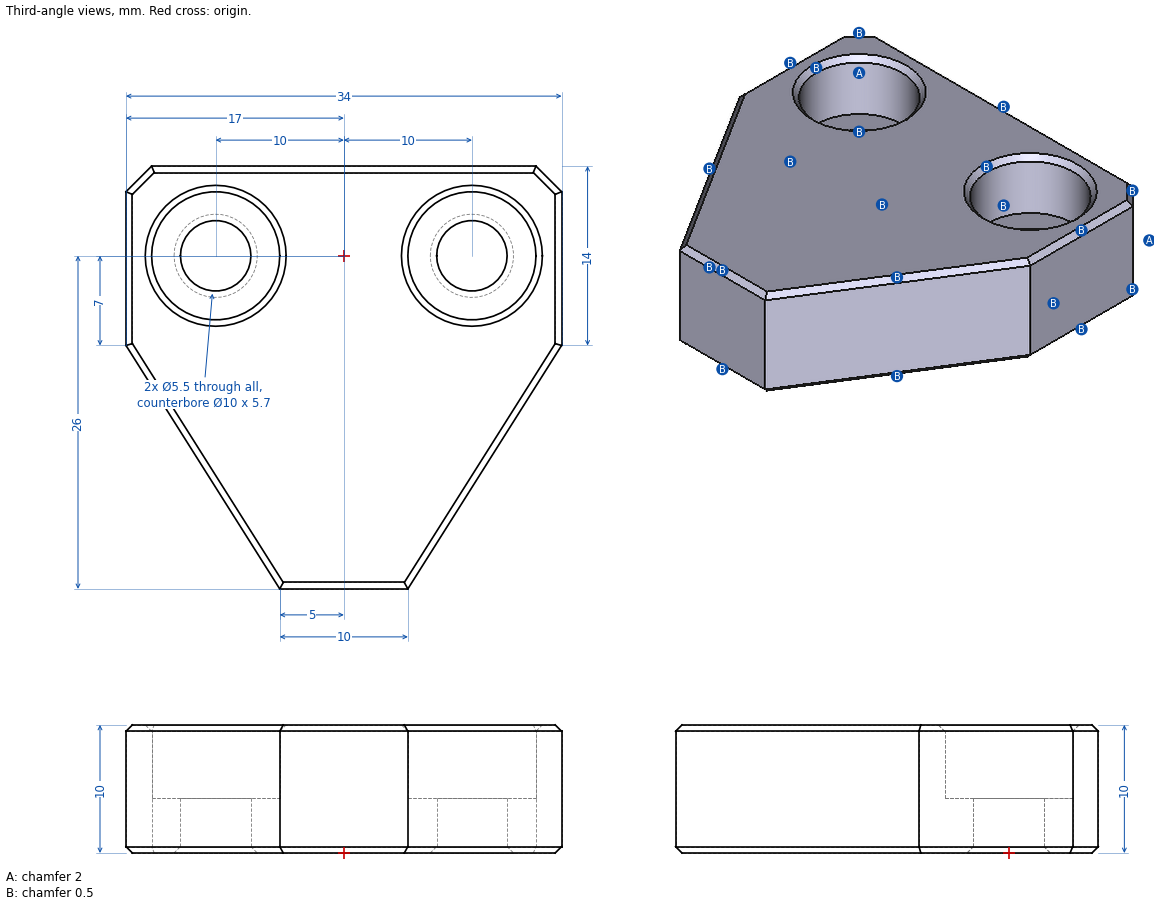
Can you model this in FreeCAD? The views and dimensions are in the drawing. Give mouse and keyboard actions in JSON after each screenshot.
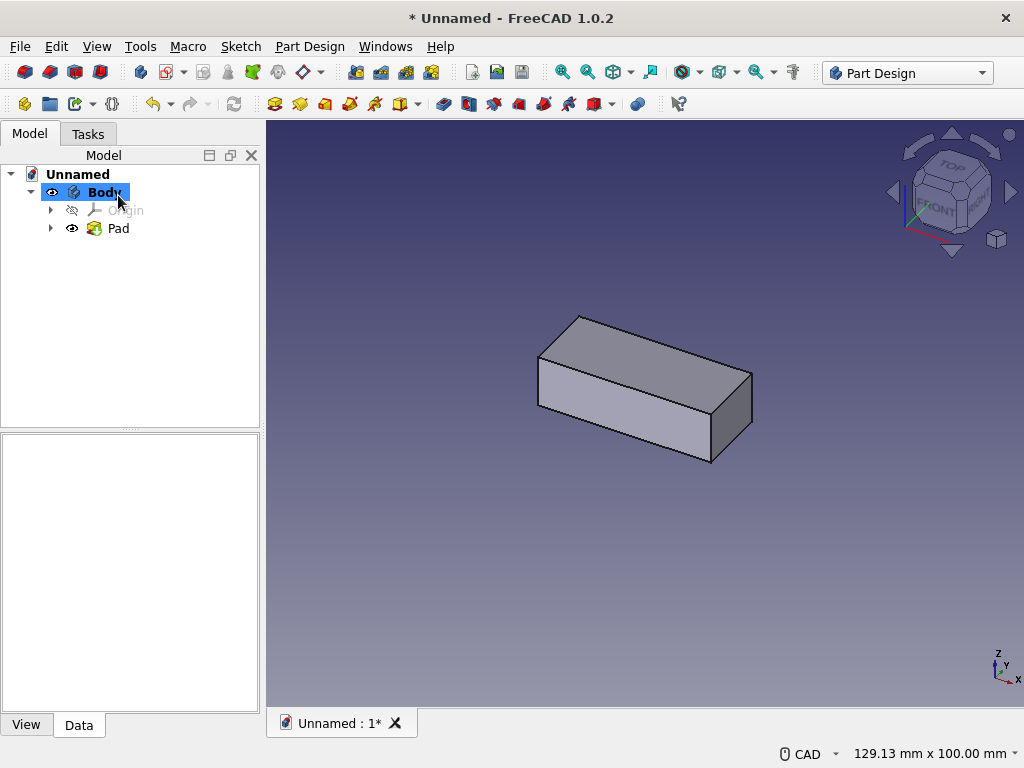
{"action": "left_click", "coordinate": [563, 72]}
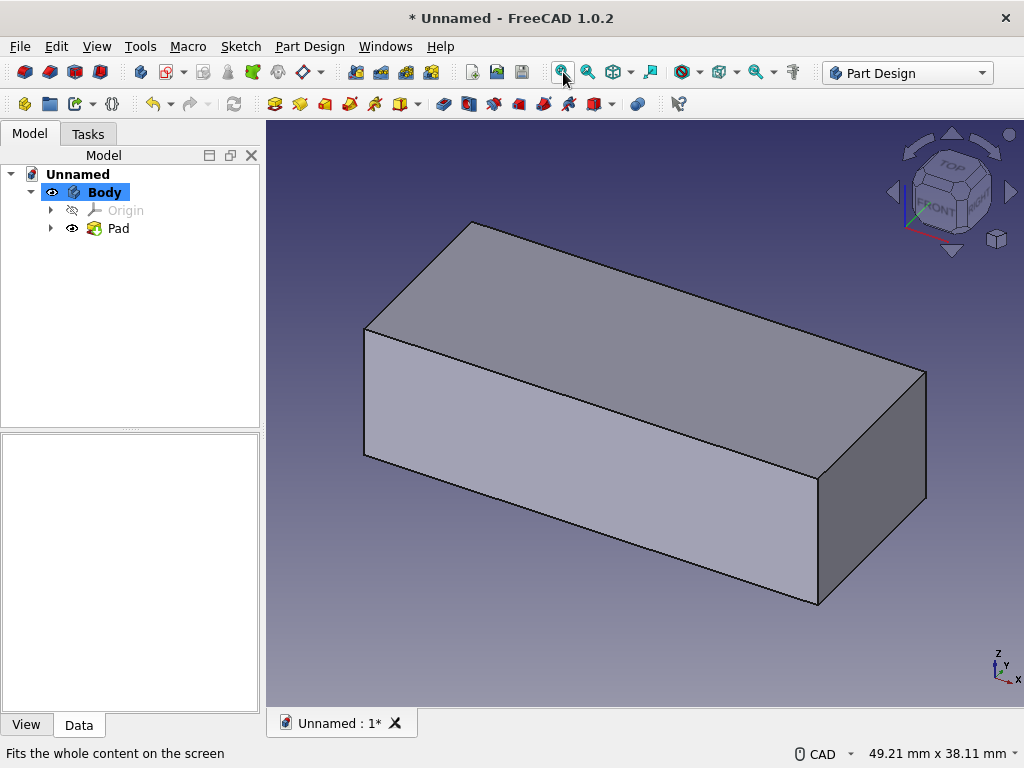
{"action": "left_click", "coordinate": [775, 392]}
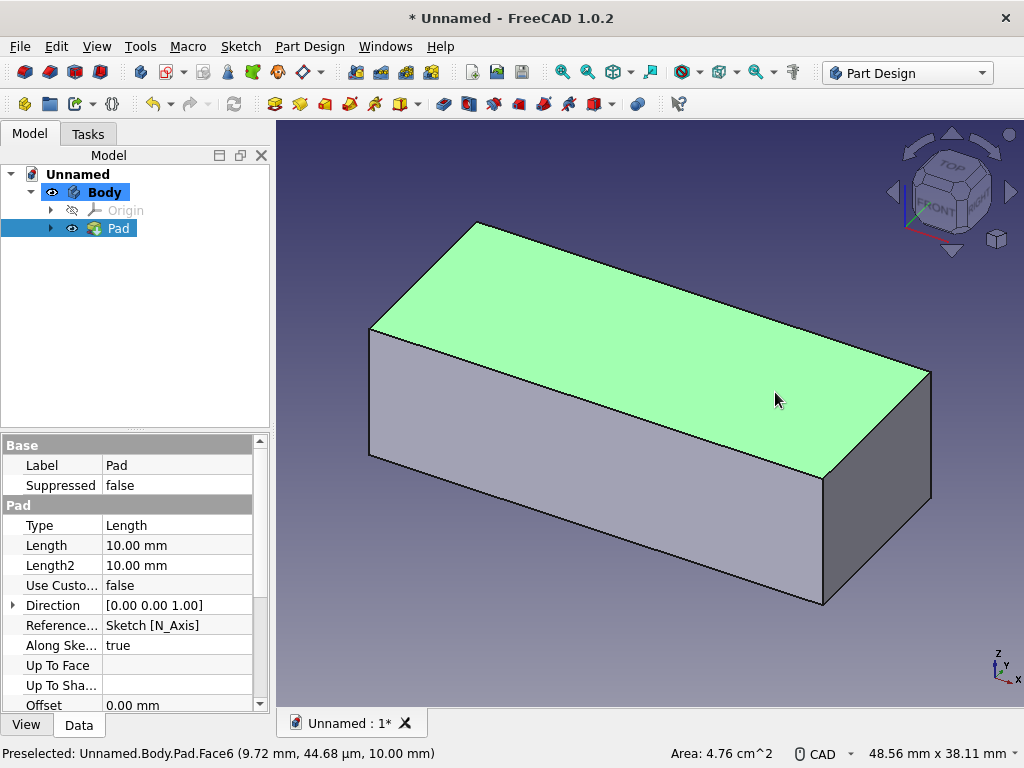
{"action": "left_click", "coordinate": [166, 72]}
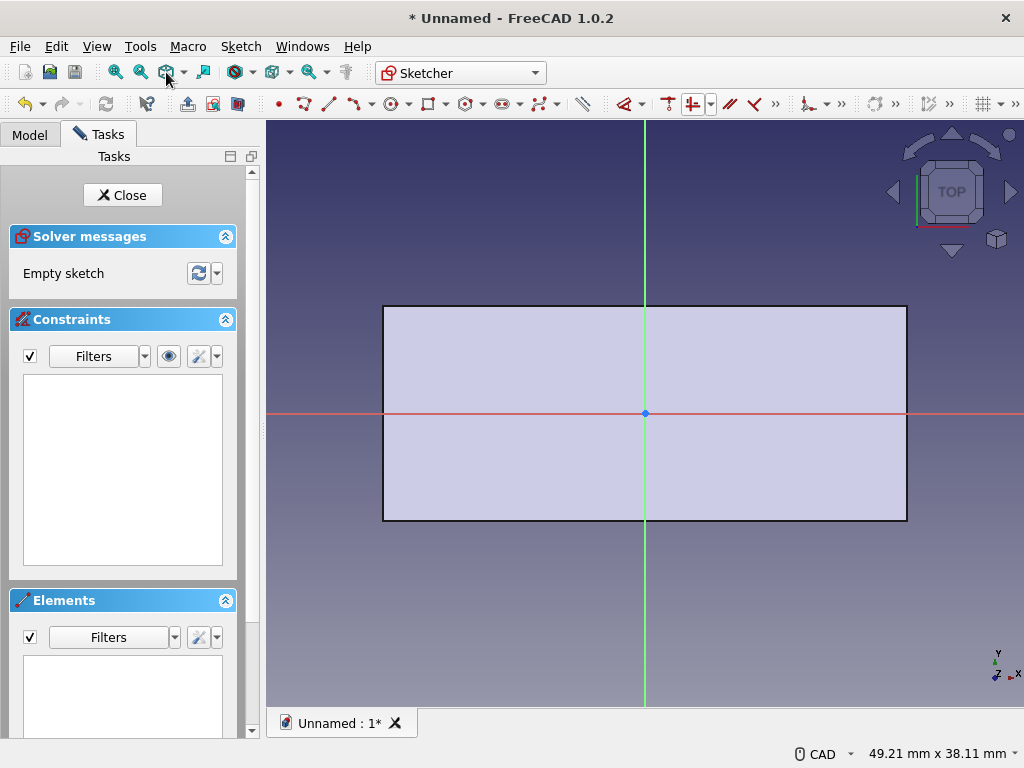
{"action": "scroll", "coordinate": [294, 413], "scroll_direction": "down", "scroll_amount": 1}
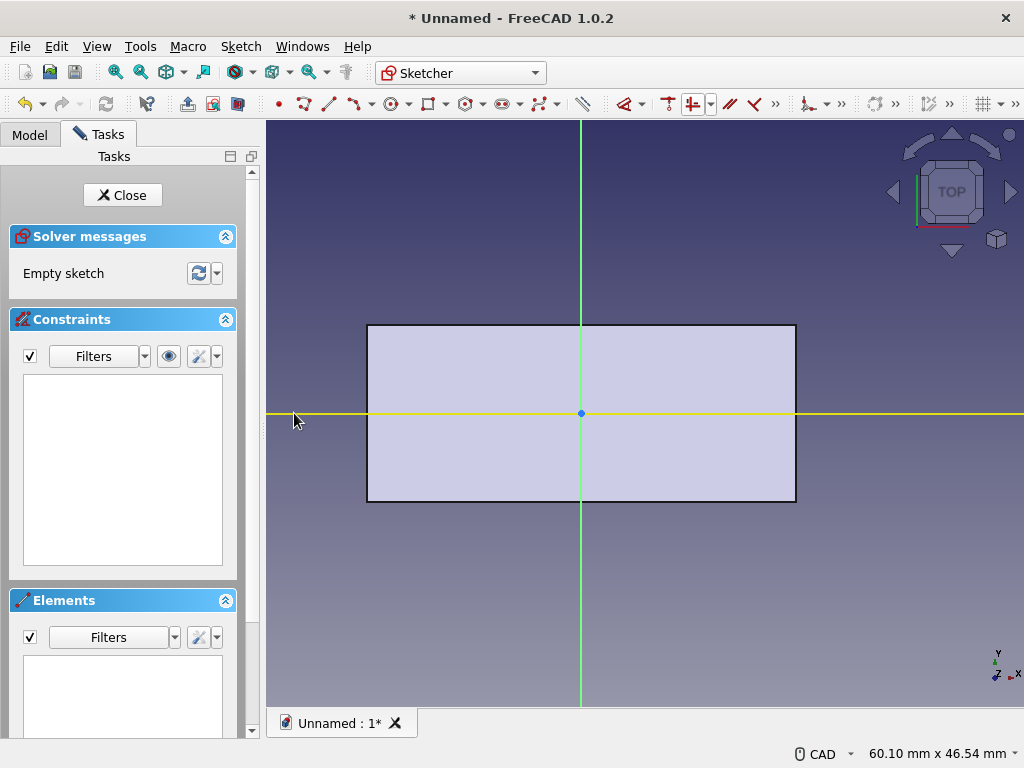
{"action": "left_click", "coordinate": [390, 104]}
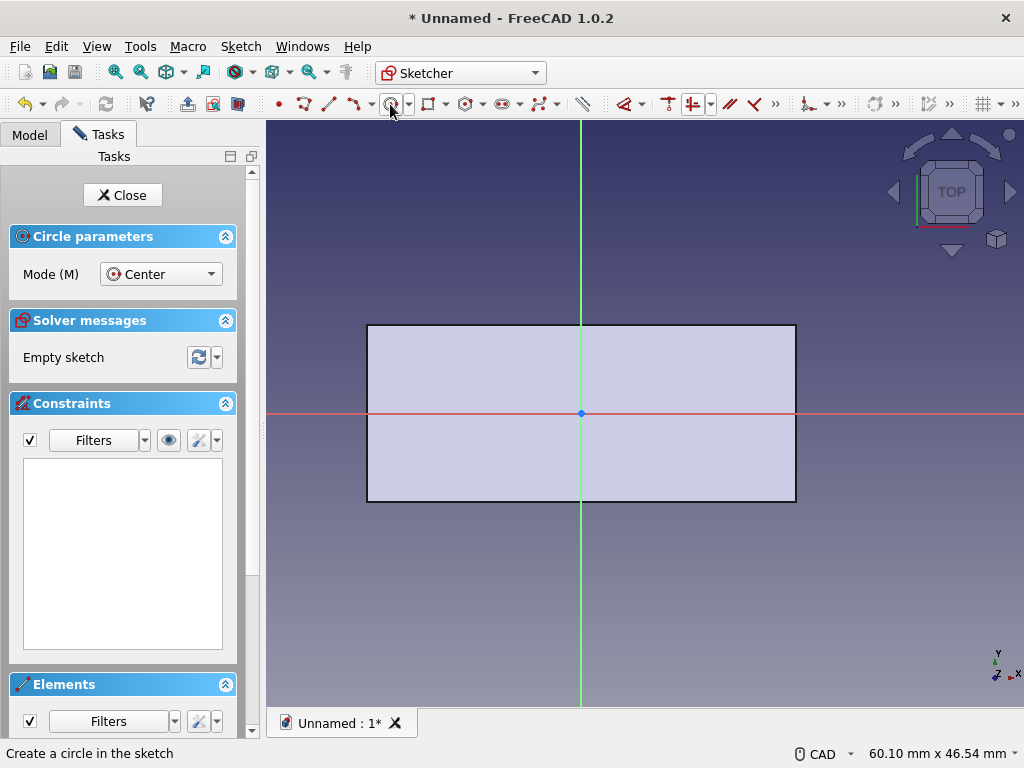
{"action": "left_click", "coordinate": [455, 414]}
{"action": "mouse_move", "coordinate": [480, 389]}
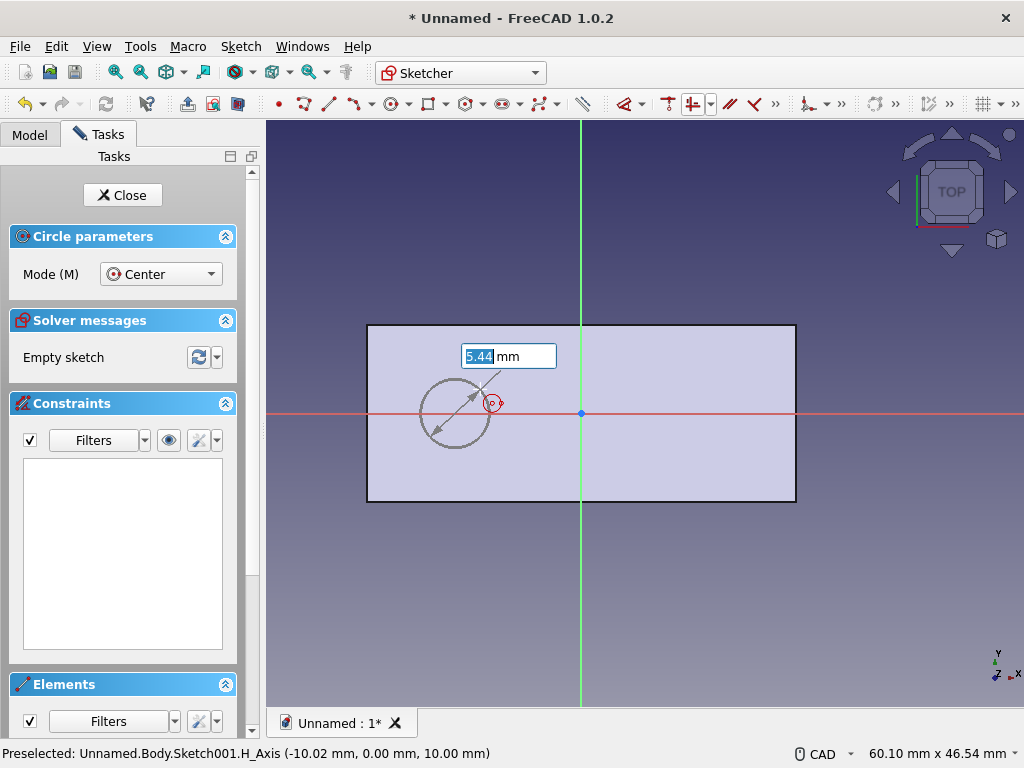
{"action": "type", "text": "5.5"}
{"action": "key", "text": "Return"}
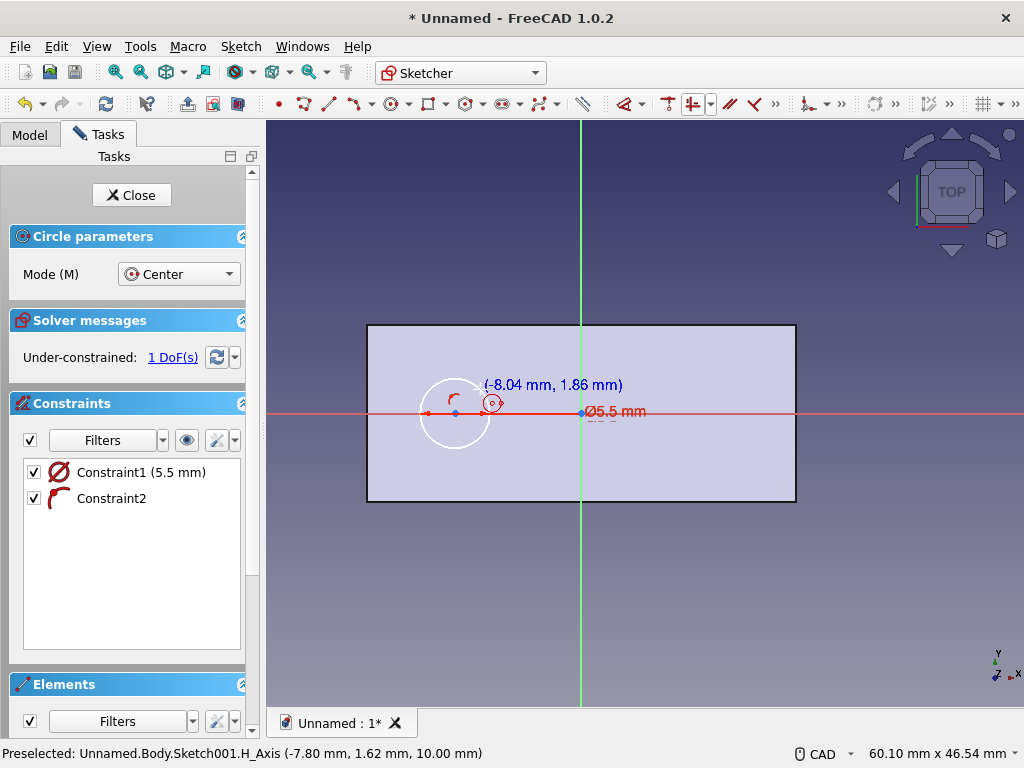
{"action": "left_click", "coordinate": [708, 414]}
{"action": "mouse_move", "coordinate": [732, 389]}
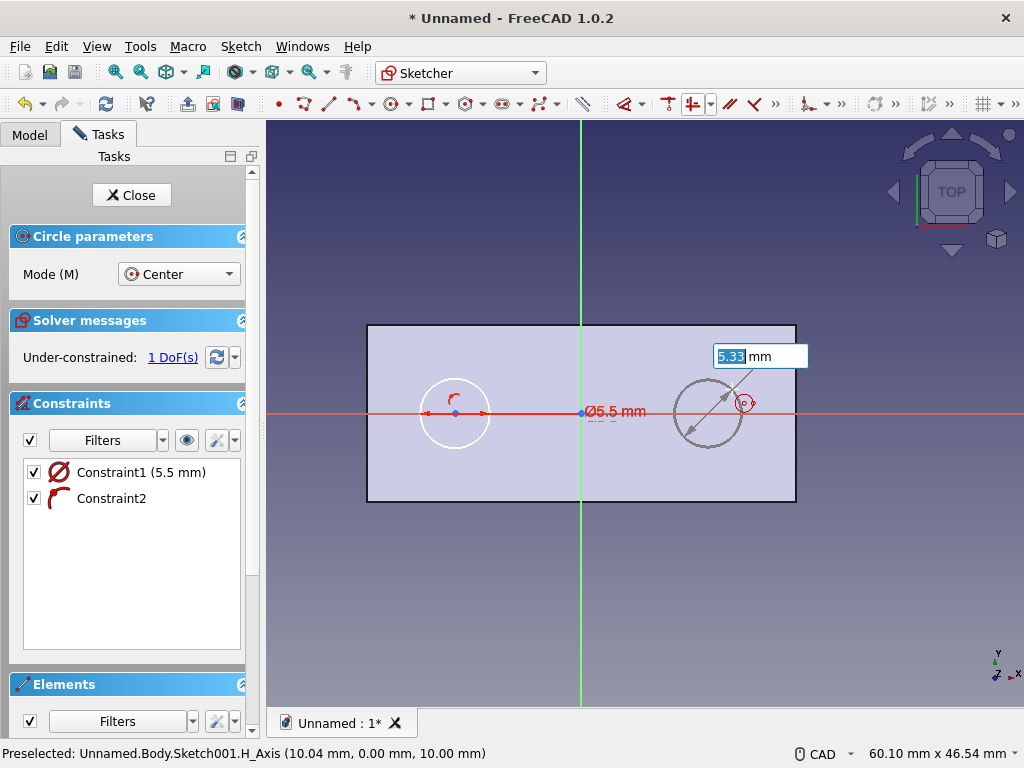
{"action": "type", "text": "5.5"}
{"action": "key", "text": "Return"}
{"action": "key", "text": "Escape"}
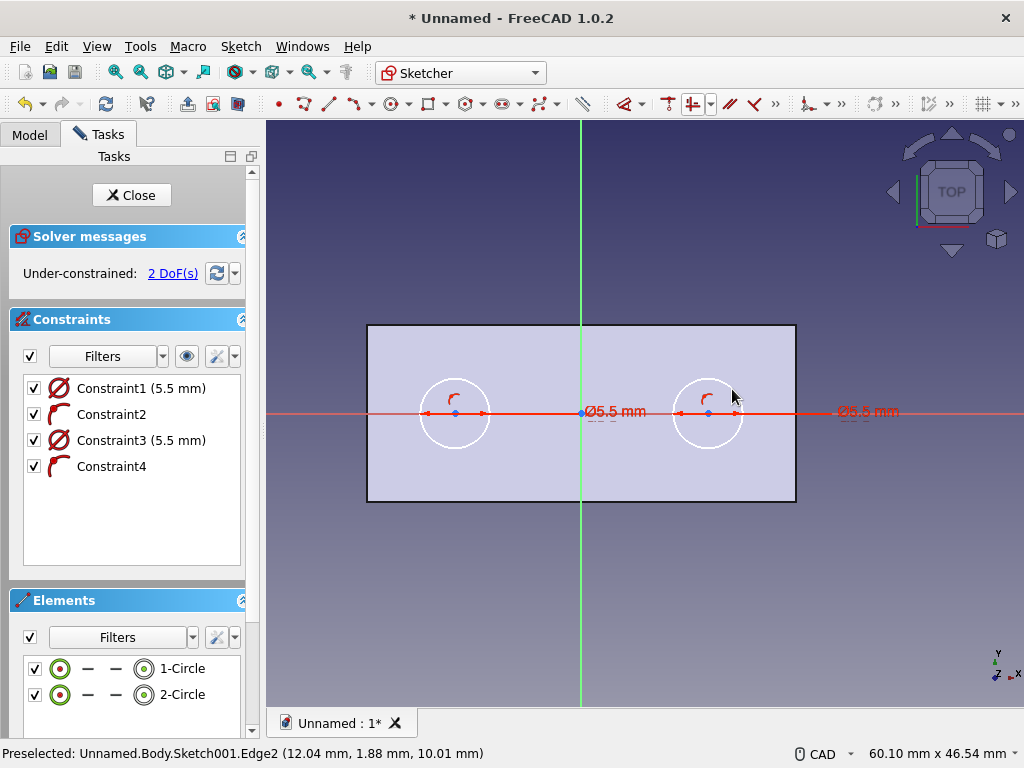
{"action": "left_click", "coordinate": [624, 104]}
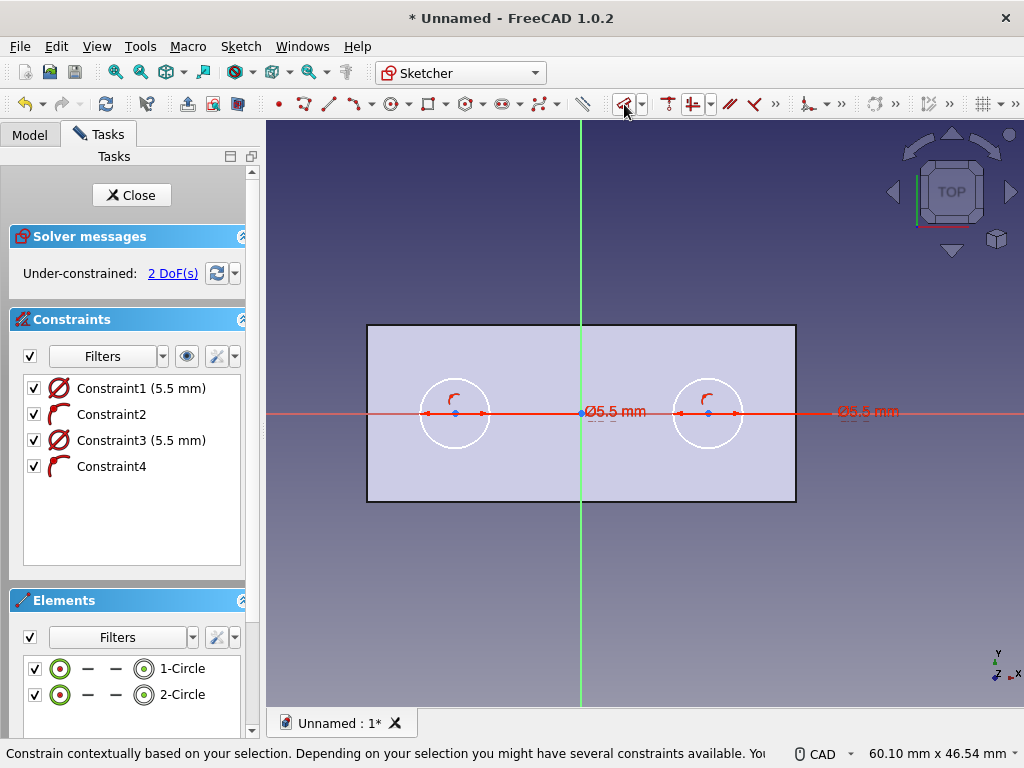
{"action": "left_click", "coordinate": [455, 414]}
{"action": "left_click", "coordinate": [518, 448]}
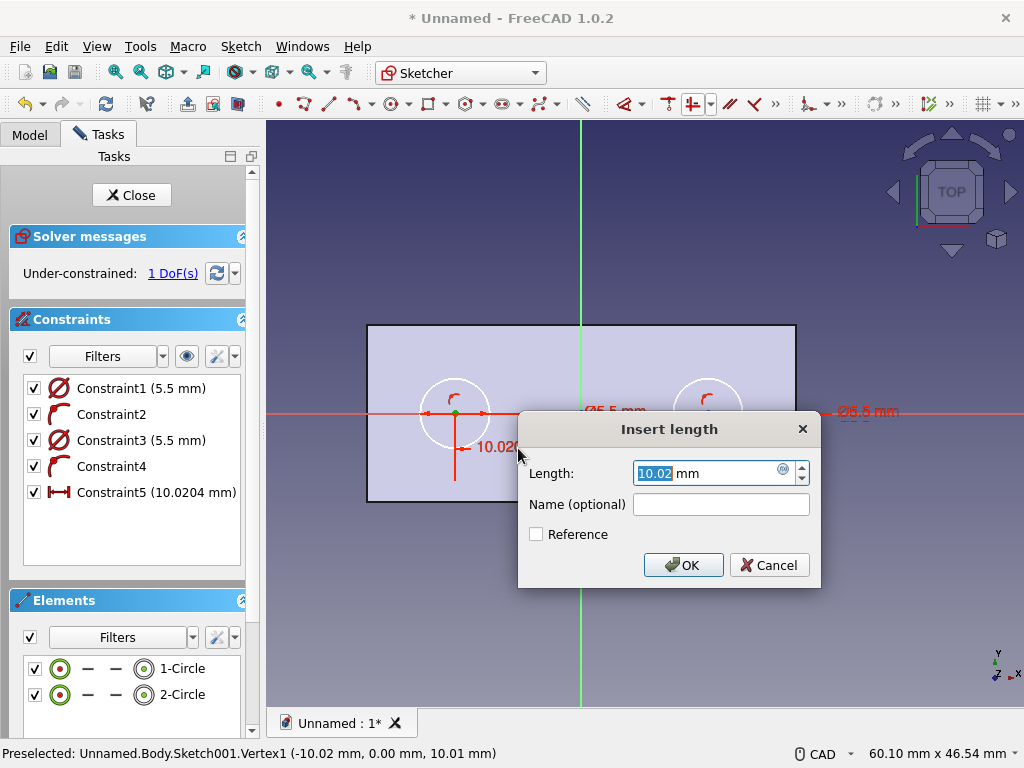
{"action": "type", "text": "10"}
{"action": "key", "text": "Return"}